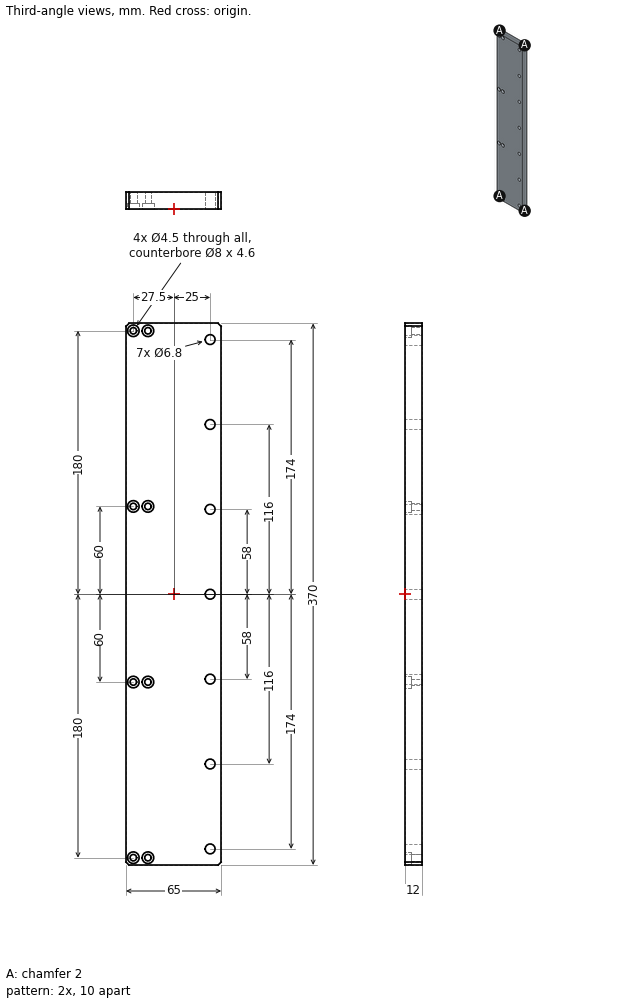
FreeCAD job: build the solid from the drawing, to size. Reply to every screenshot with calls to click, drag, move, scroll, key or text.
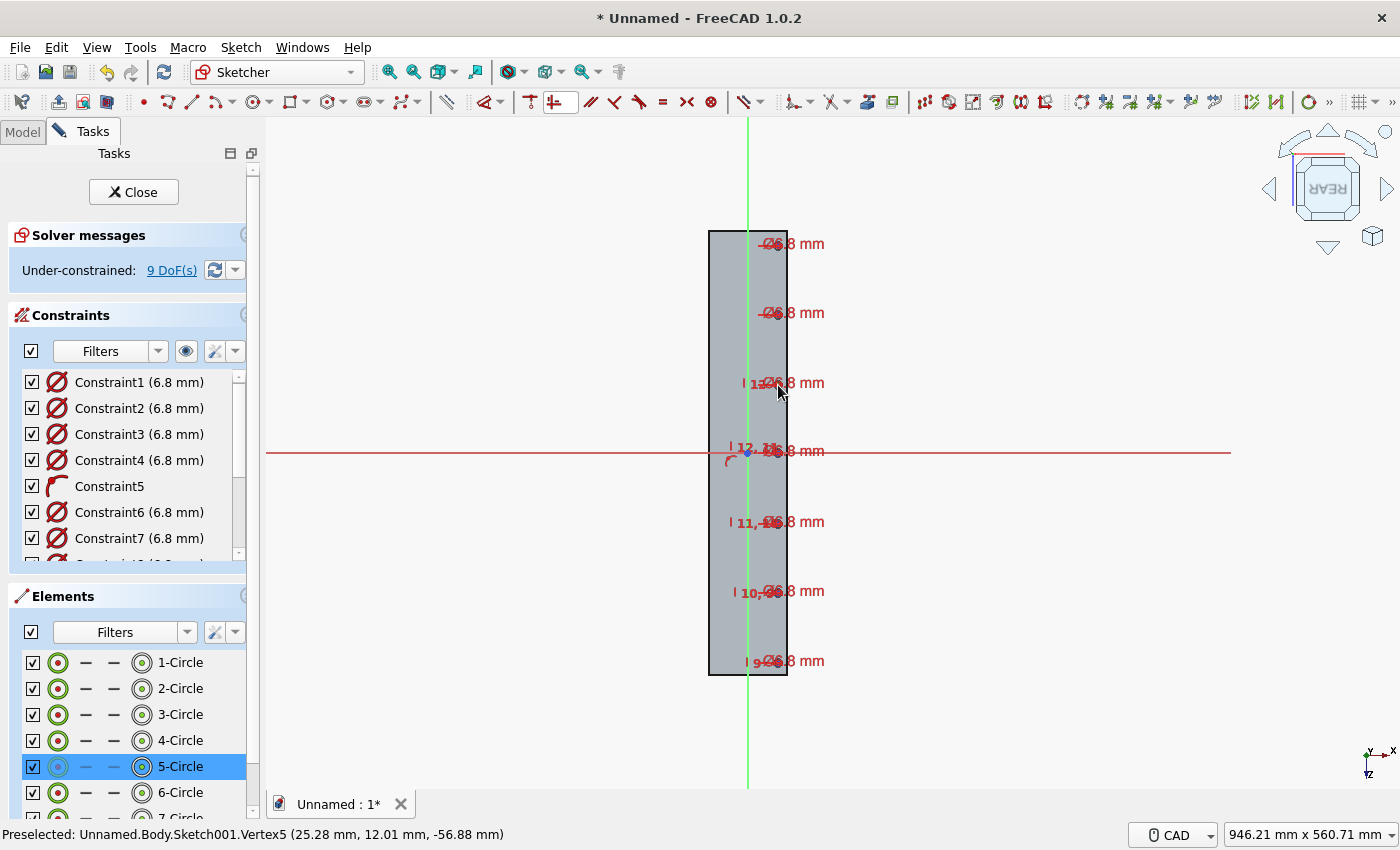
click(778, 315)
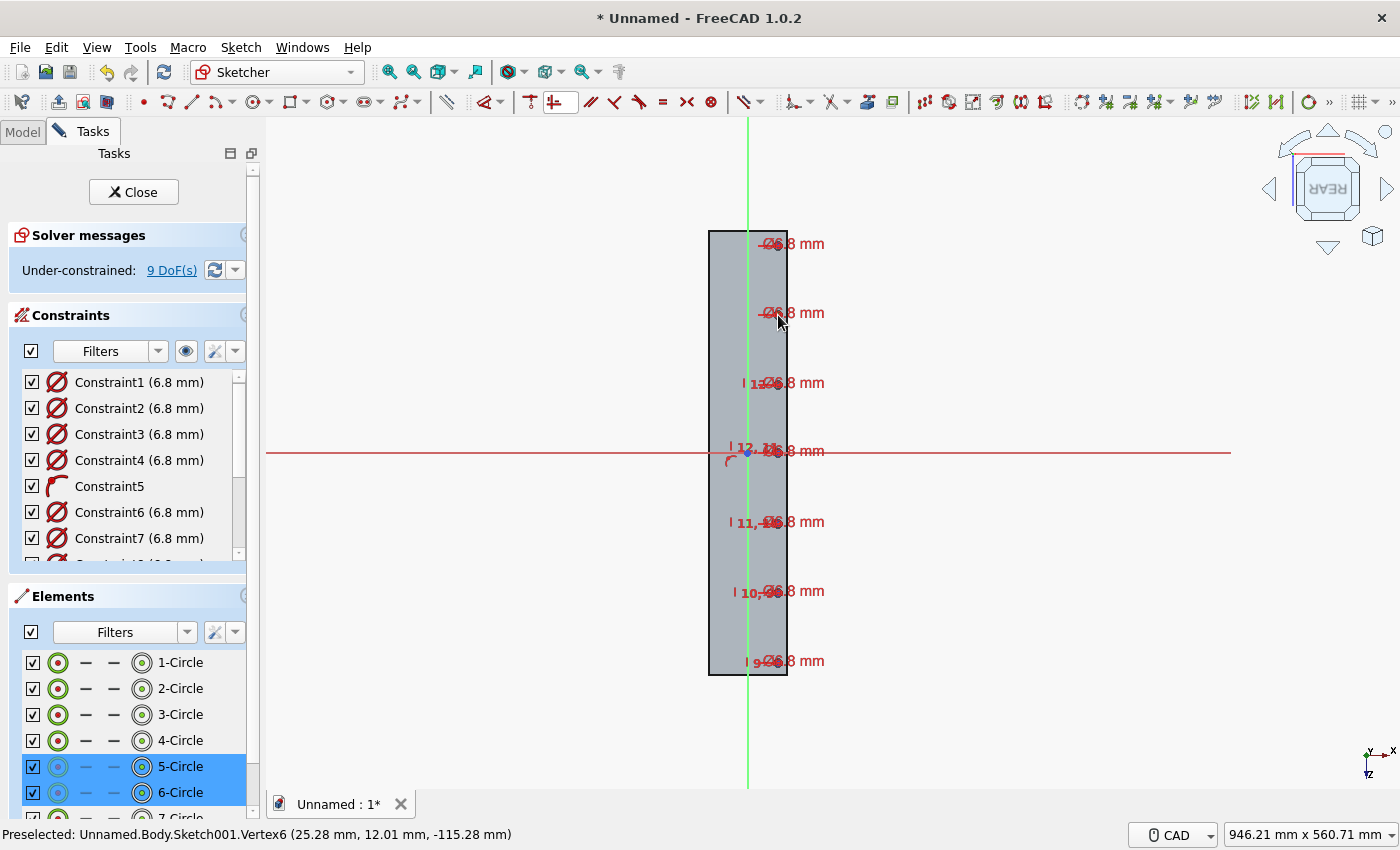
key(v)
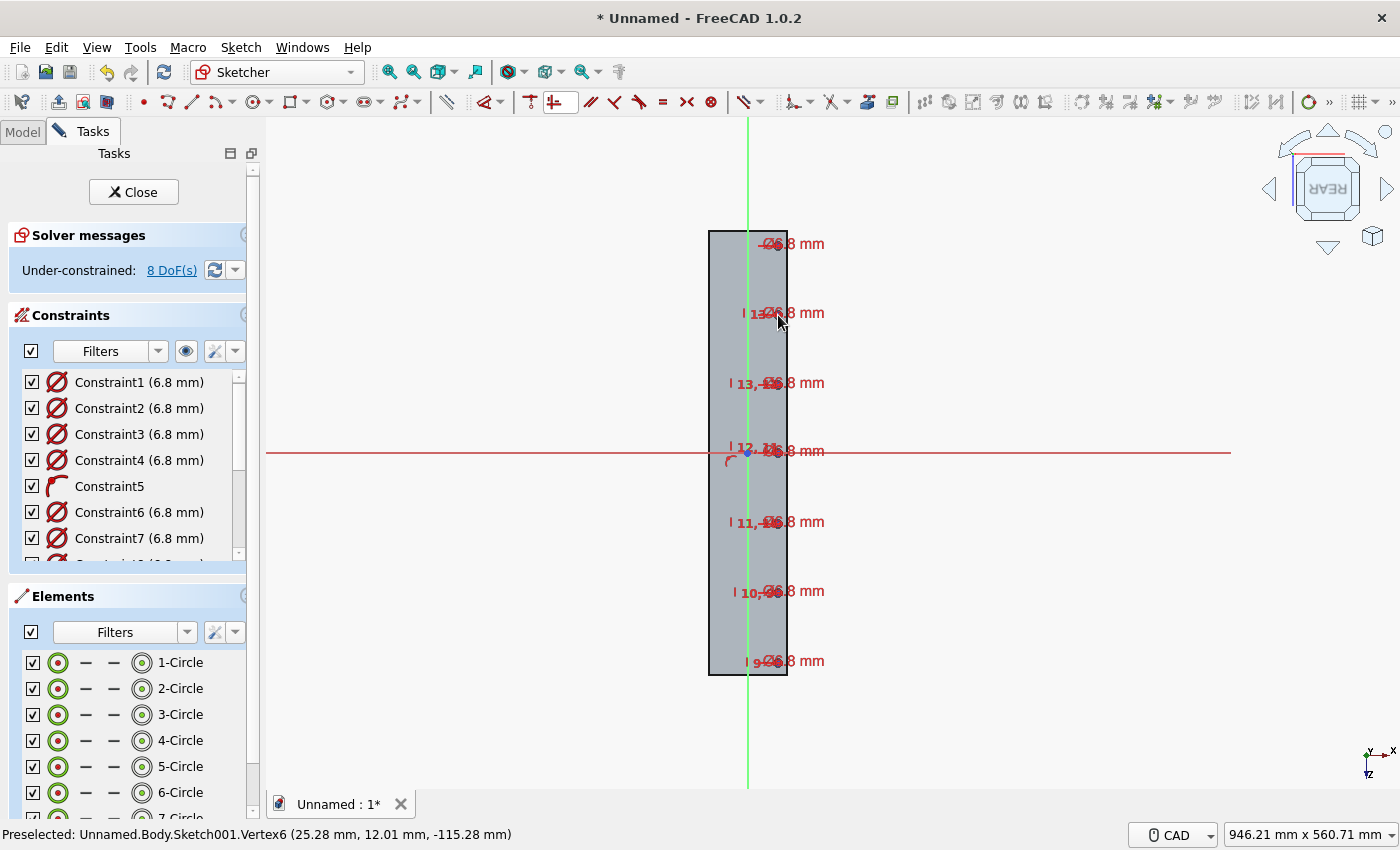
click(778, 315)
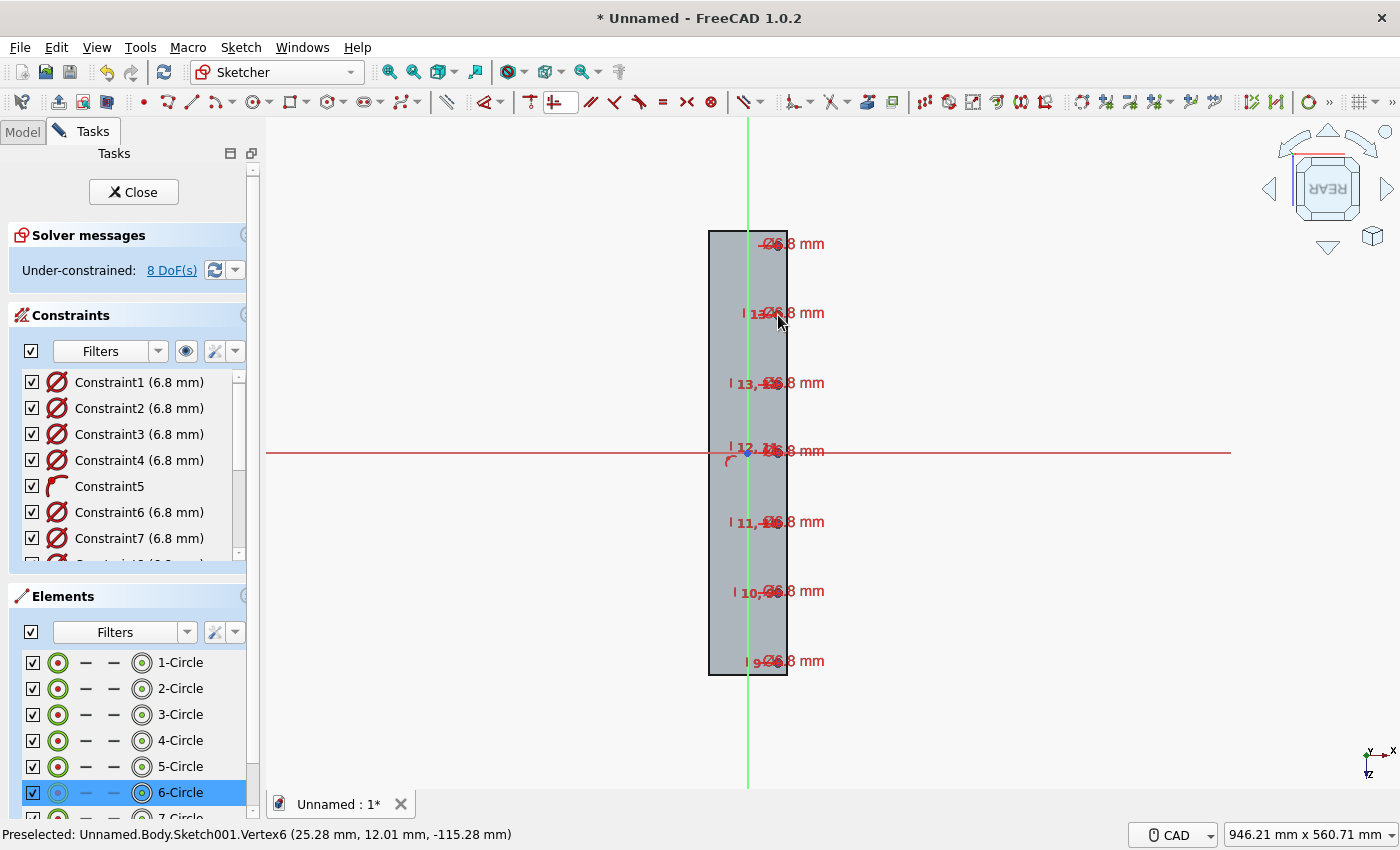
click(778, 246)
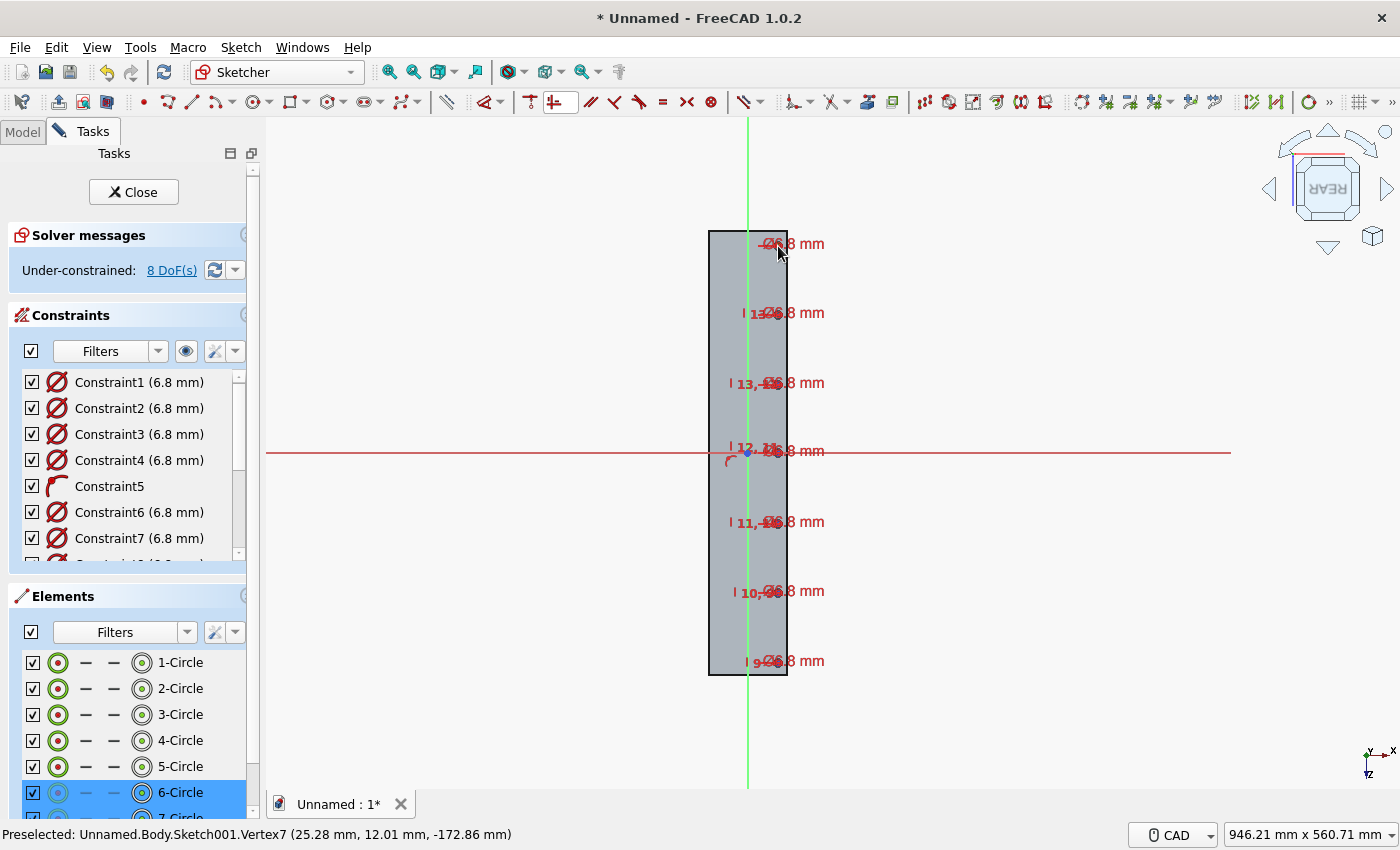
key(v)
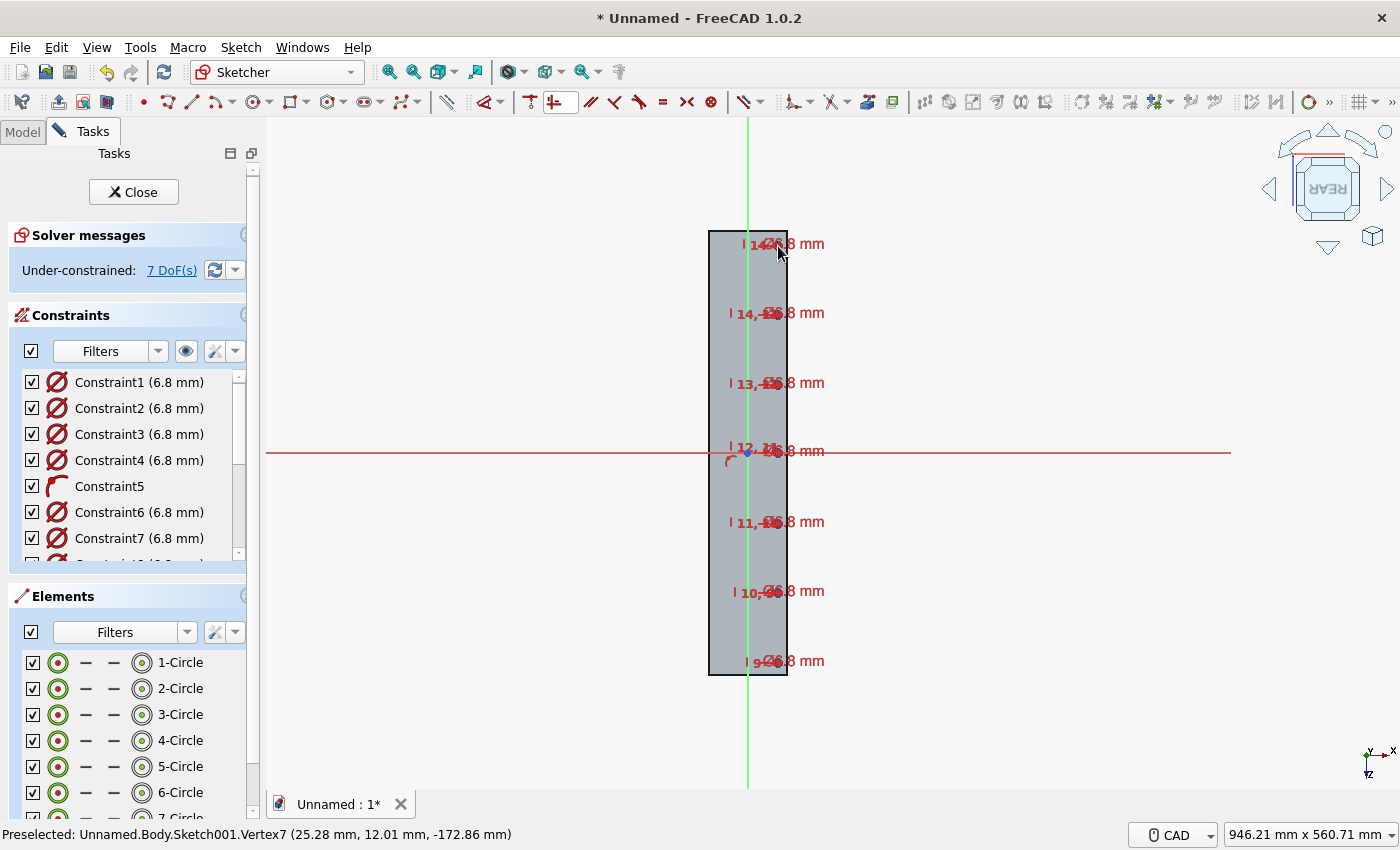
key(d)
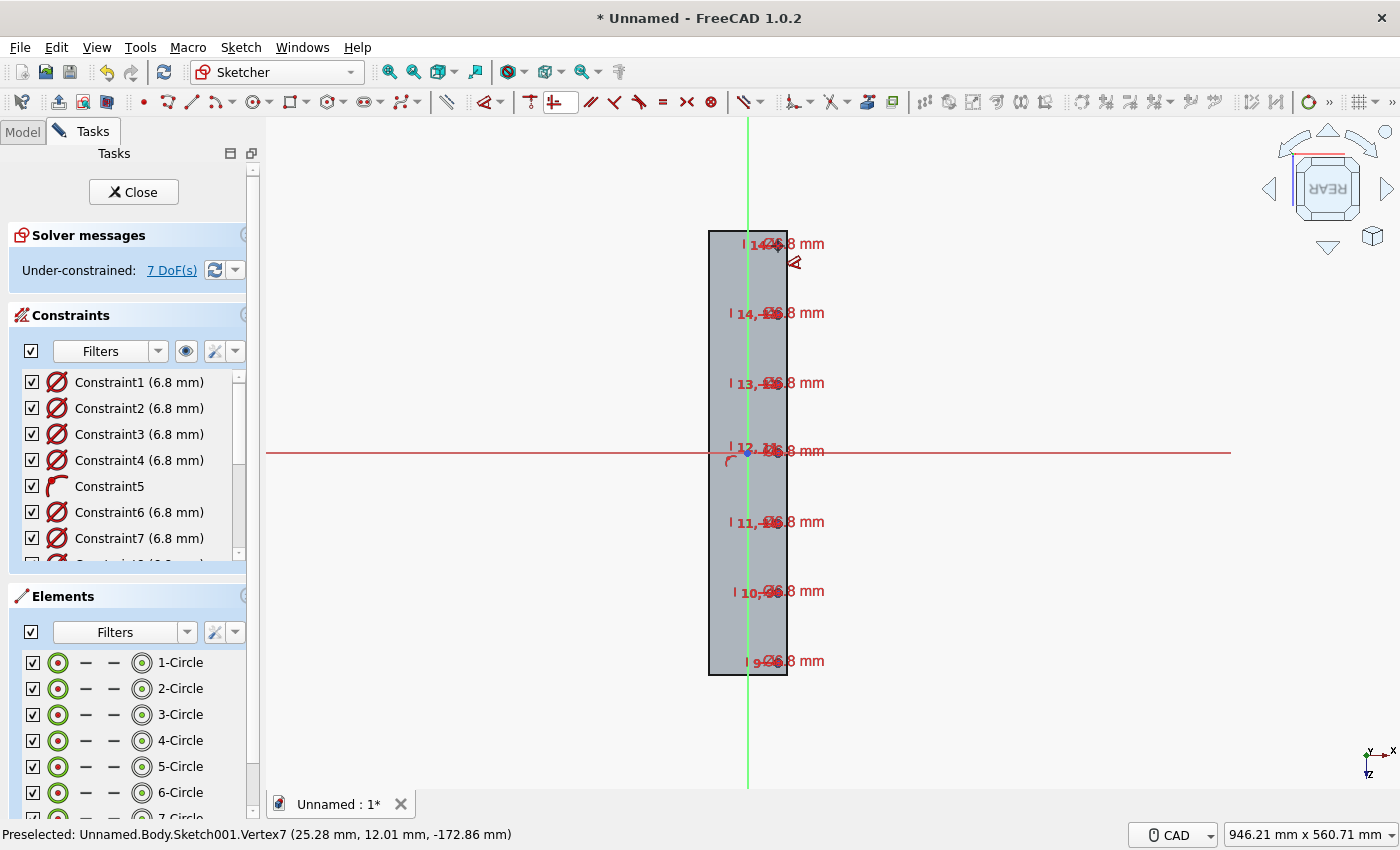
scroll(778, 663, up, 2)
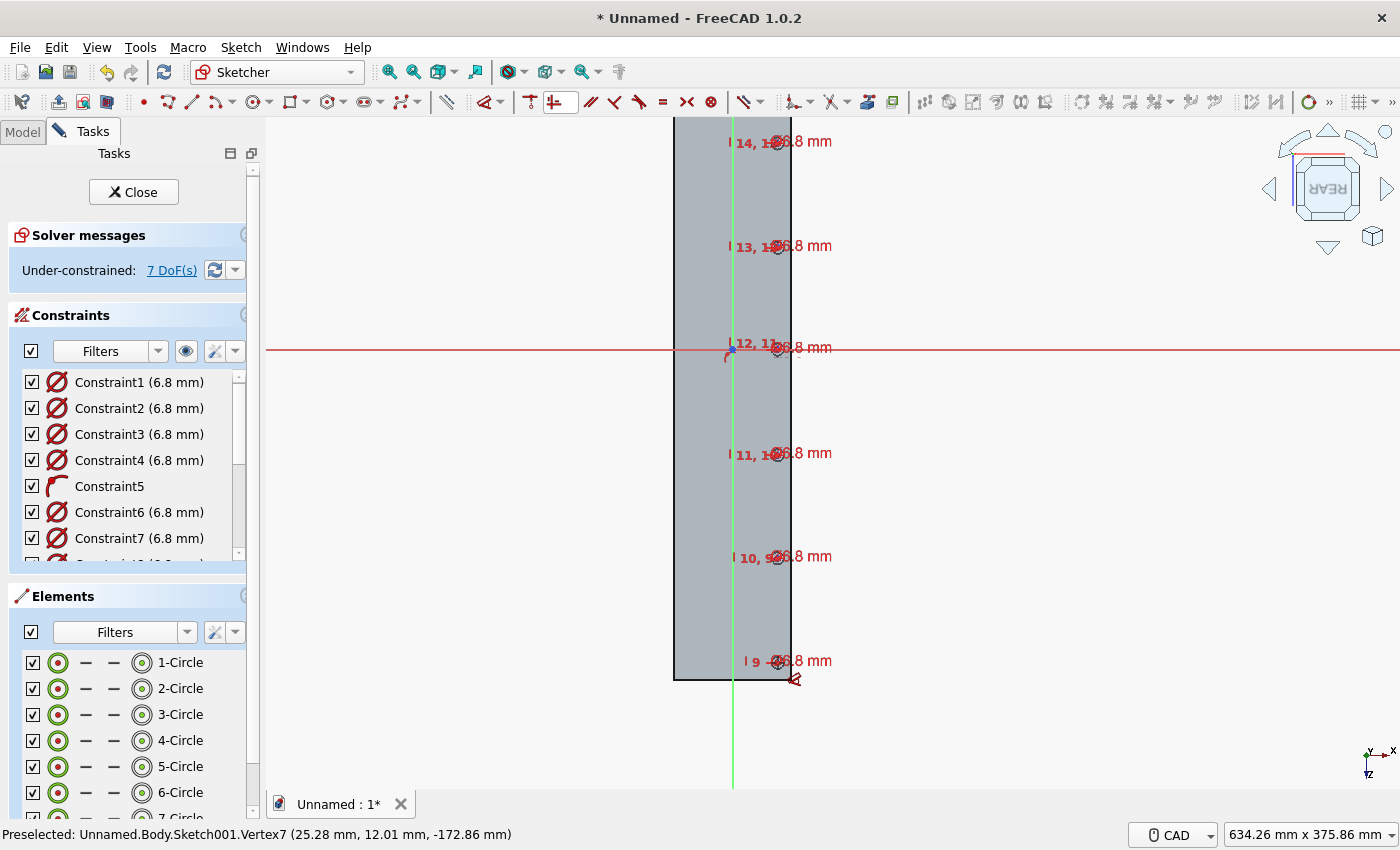
click(778, 663)
click(755, 697)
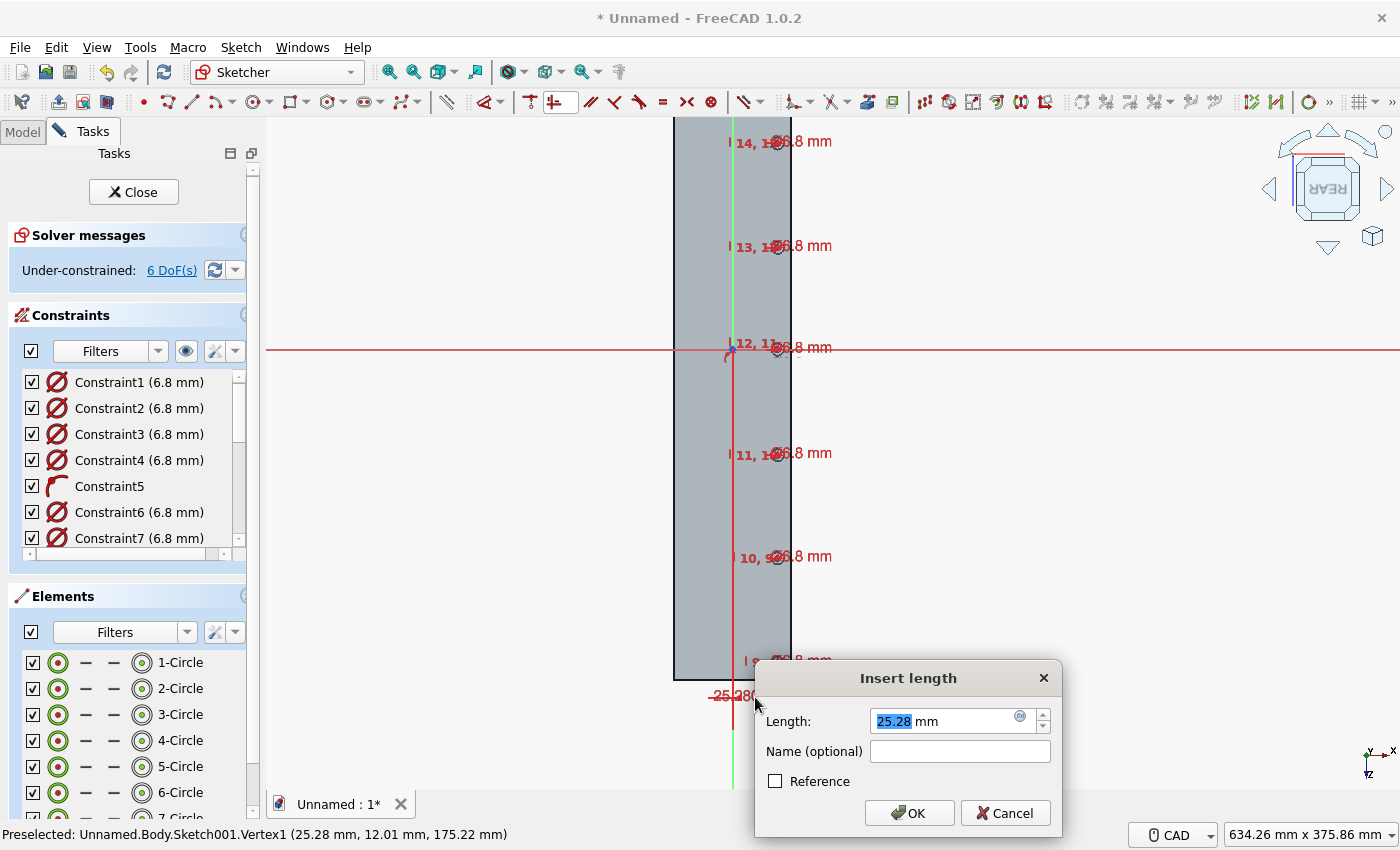
text(25)
key(Return)